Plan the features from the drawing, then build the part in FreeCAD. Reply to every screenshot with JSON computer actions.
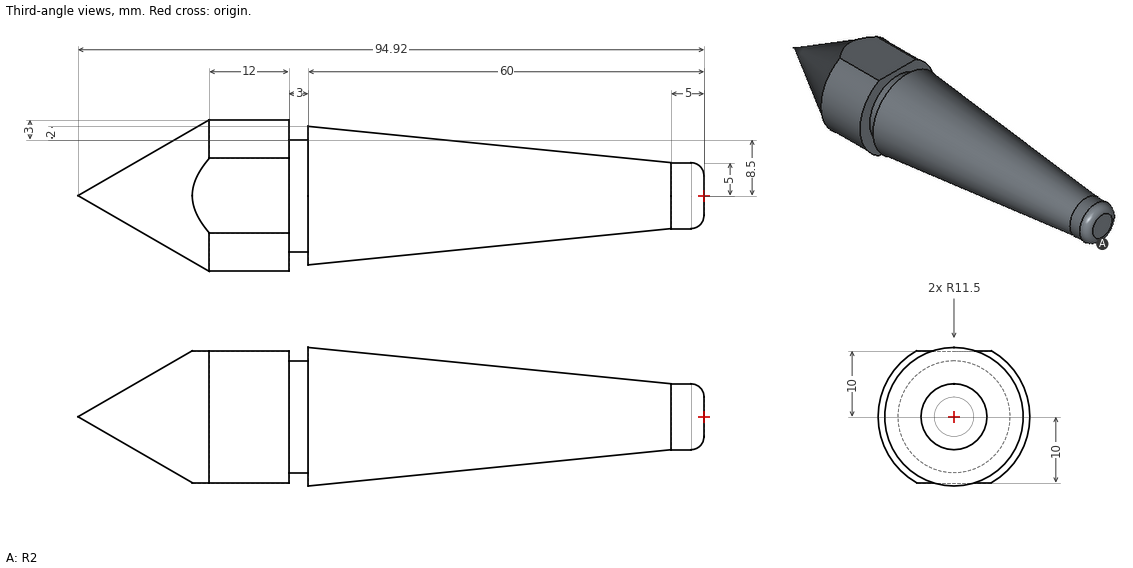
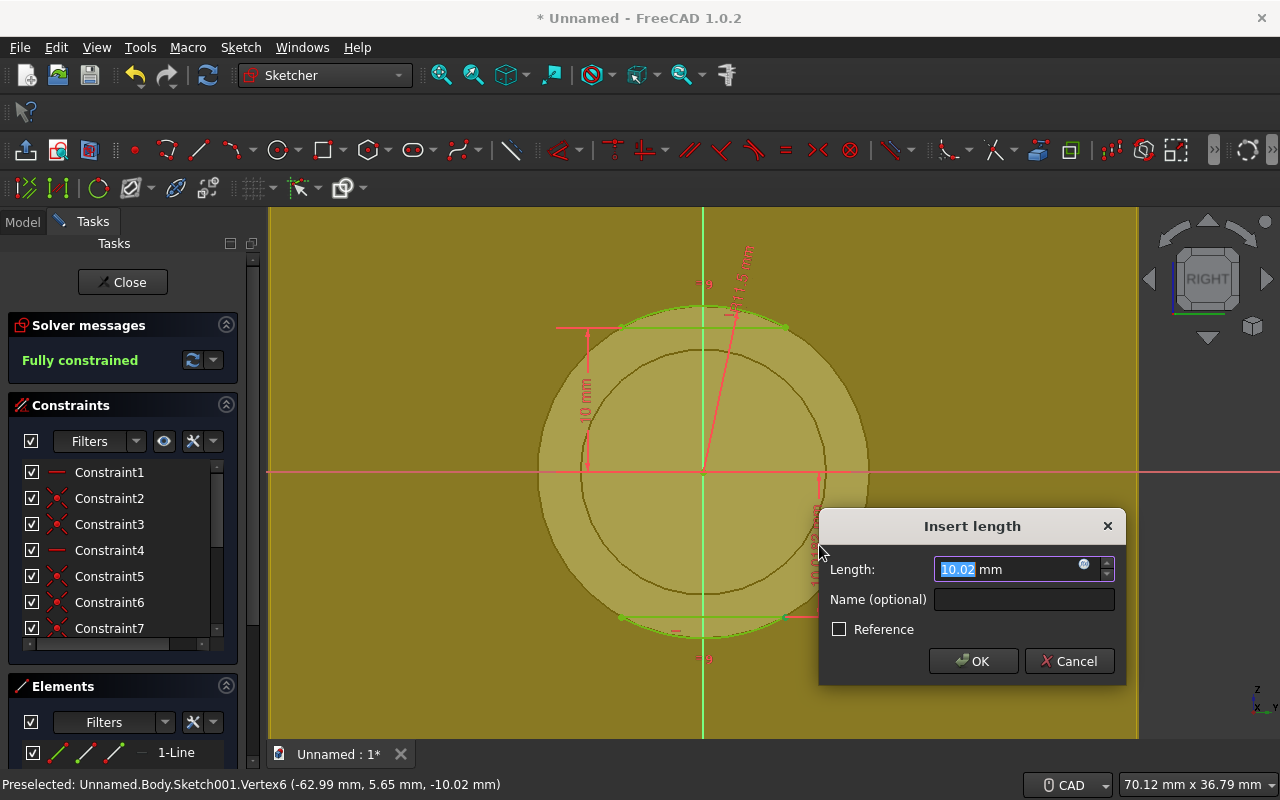
{"action": "type", "text": "10"}
{"action": "key", "text": "Return"}
{"action": "key", "text": "Escape"}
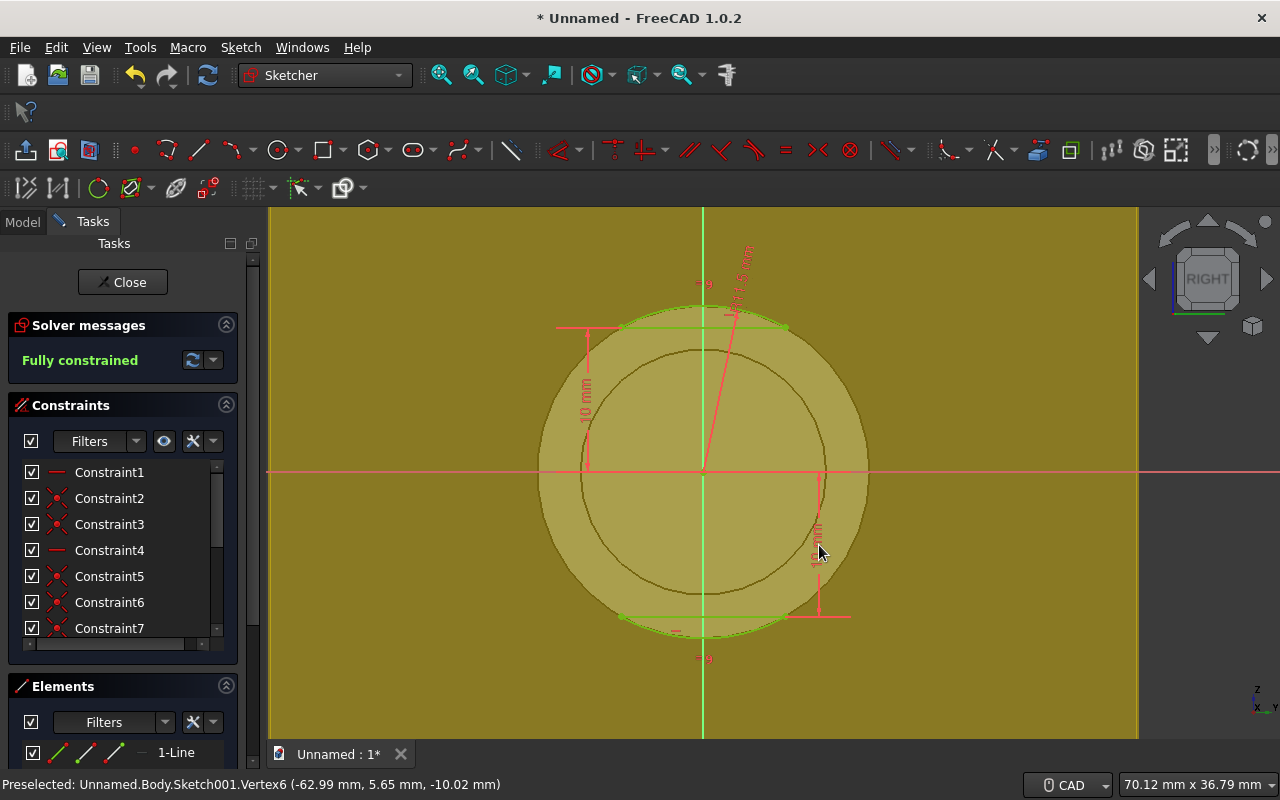
{"action": "left_click", "coordinate": [123, 282]}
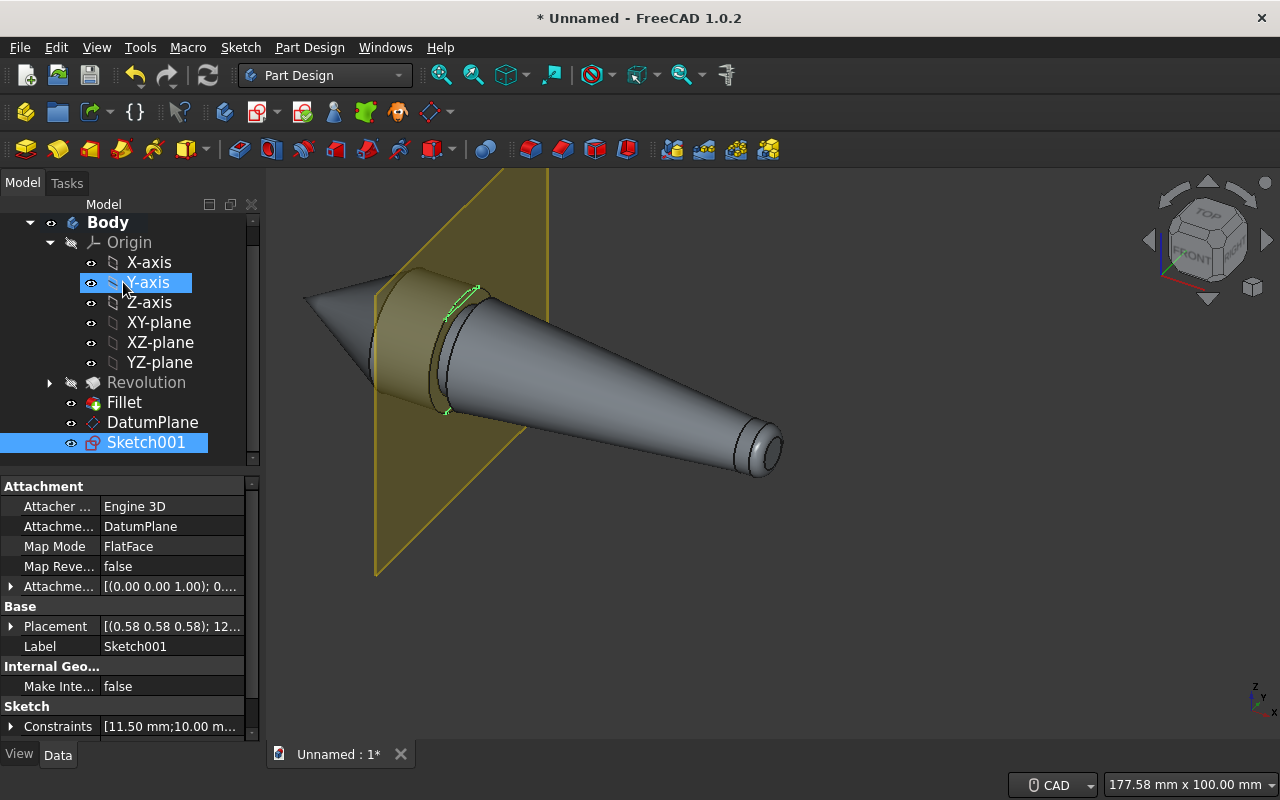
{"action": "left_click", "coordinate": [240, 150]}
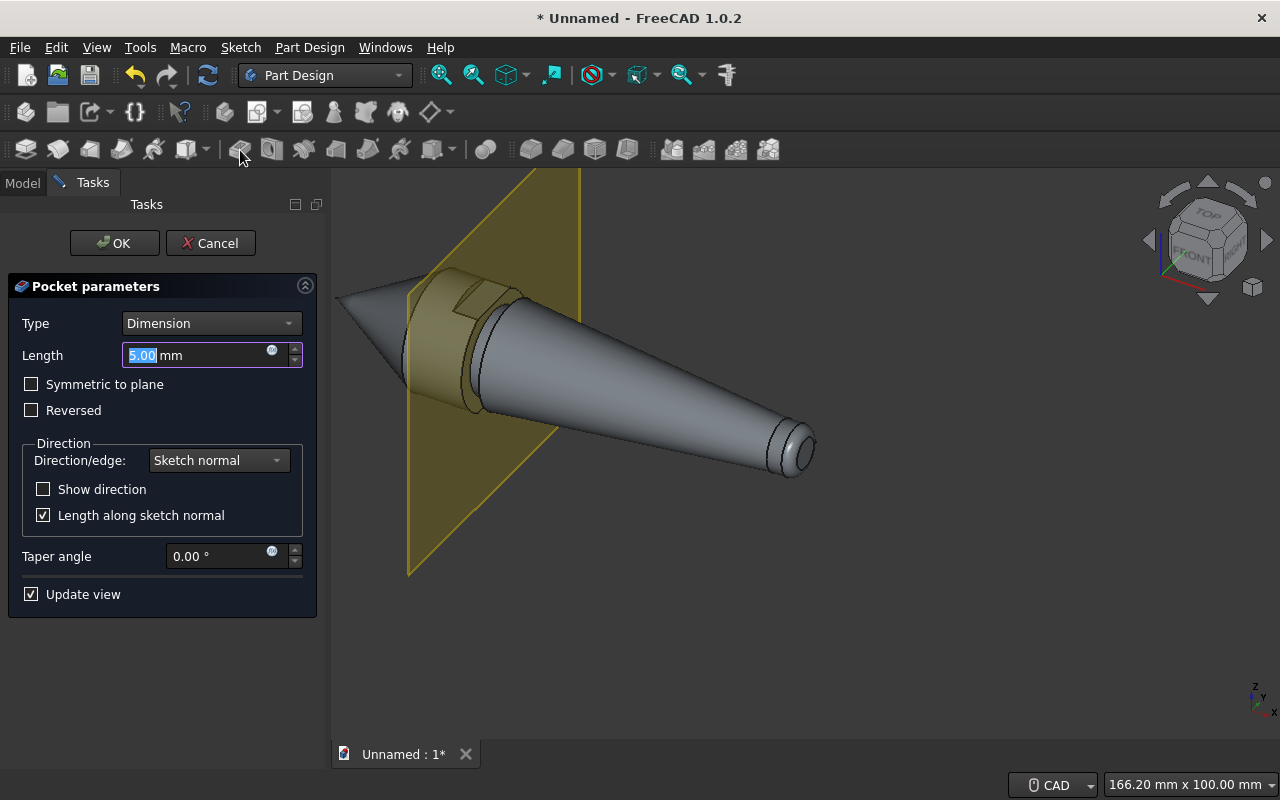
{"action": "left_click", "coordinate": [212, 324]}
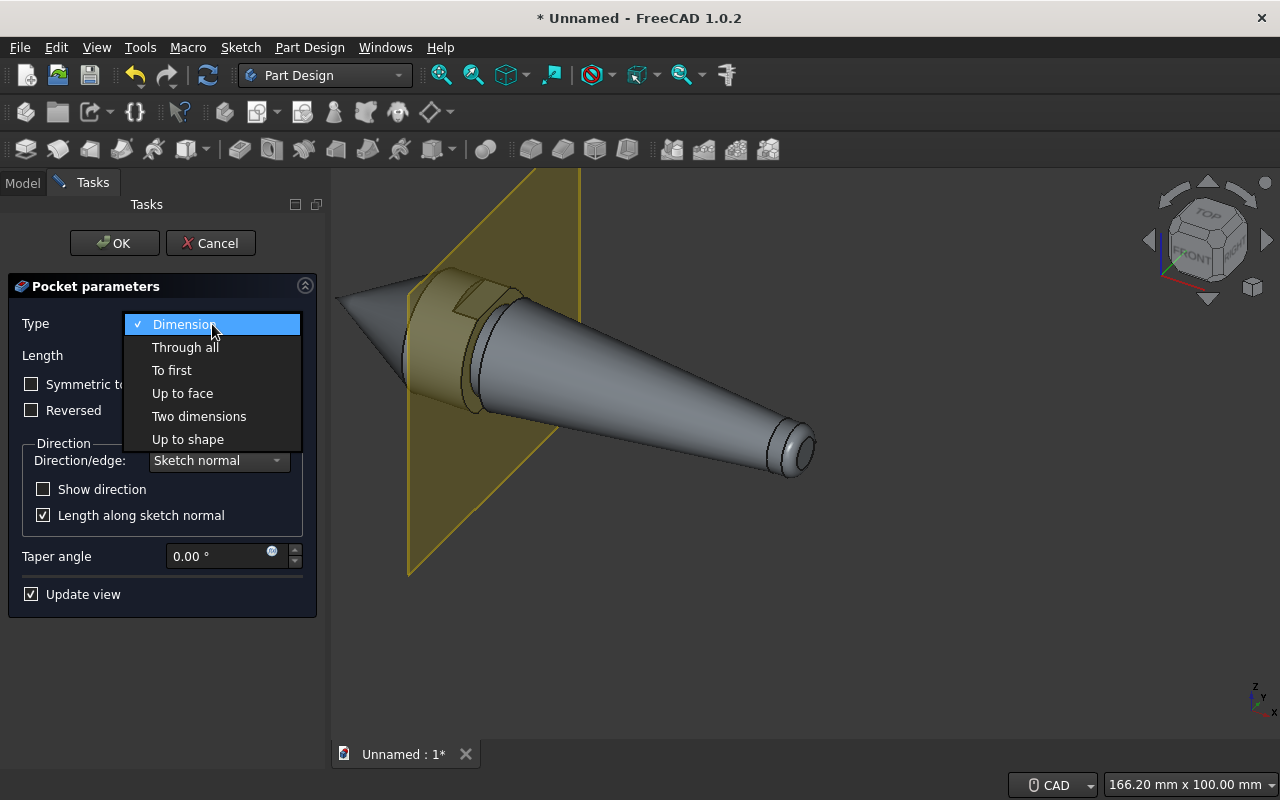
{"action": "left_click", "coordinate": [212, 348]}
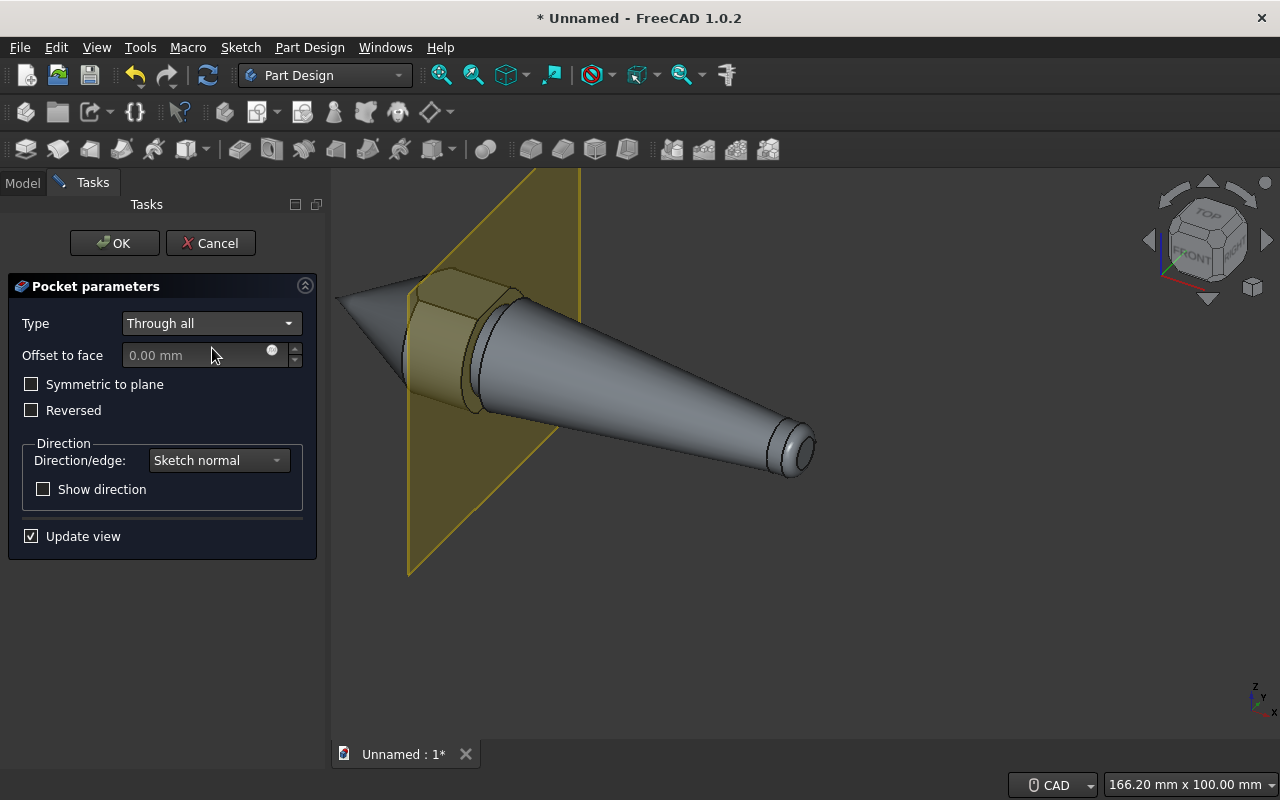
{"action": "left_click", "coordinate": [115, 243]}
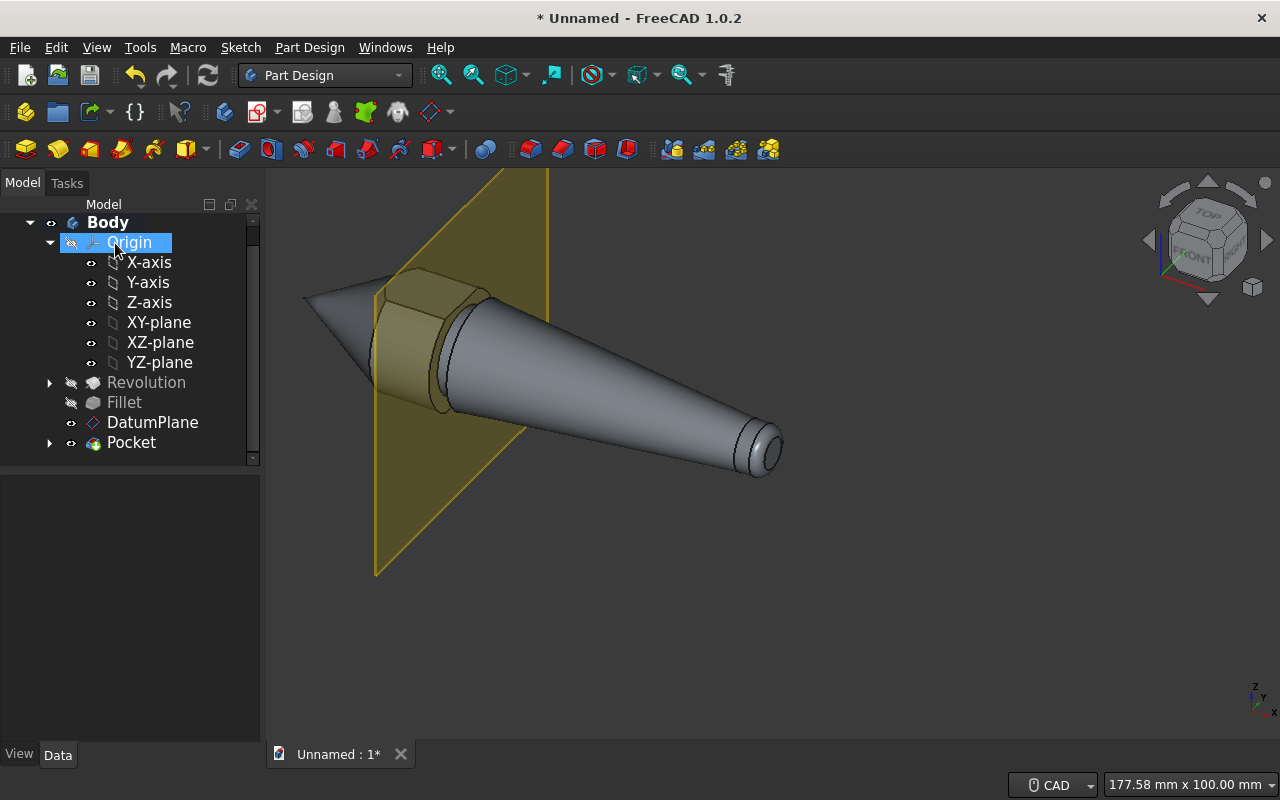
{"action": "left_click", "coordinate": [116, 423]}
{"action": "key", "text": "space"}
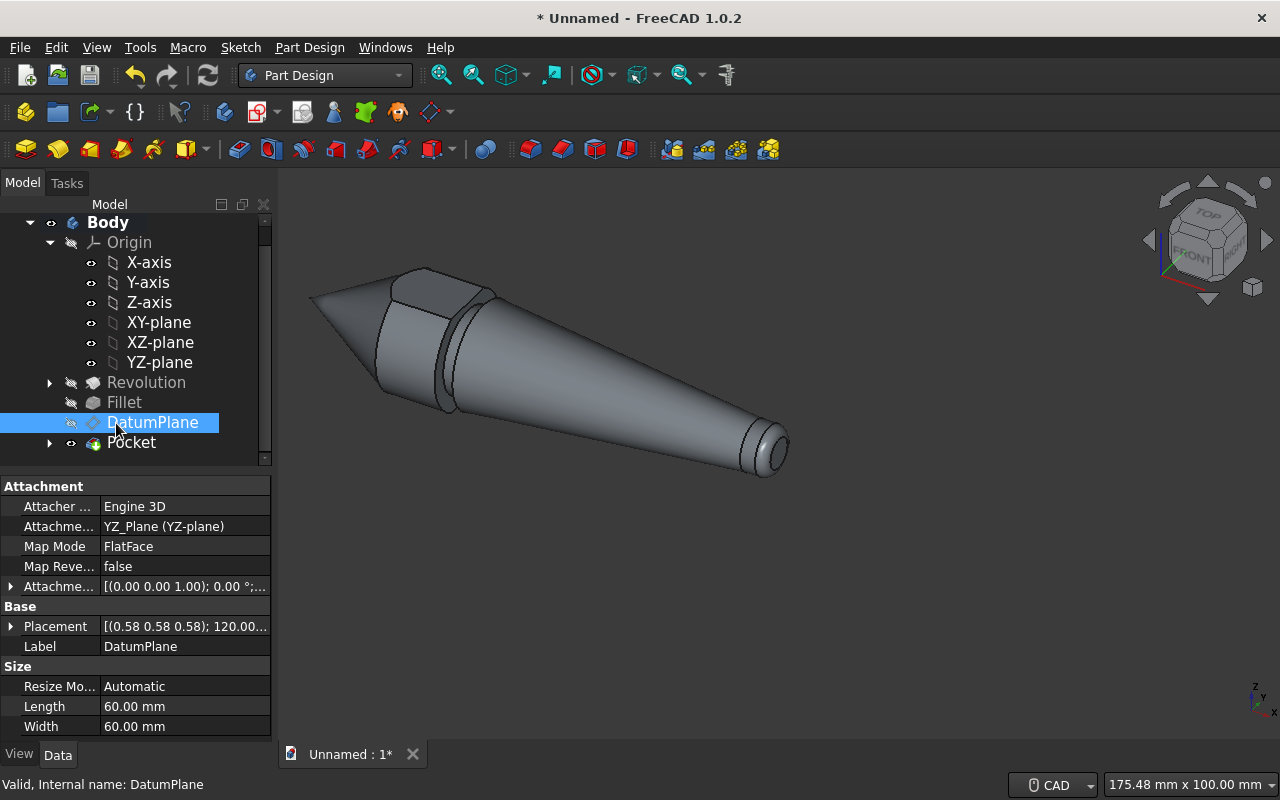
{"action": "key", "text": "0"}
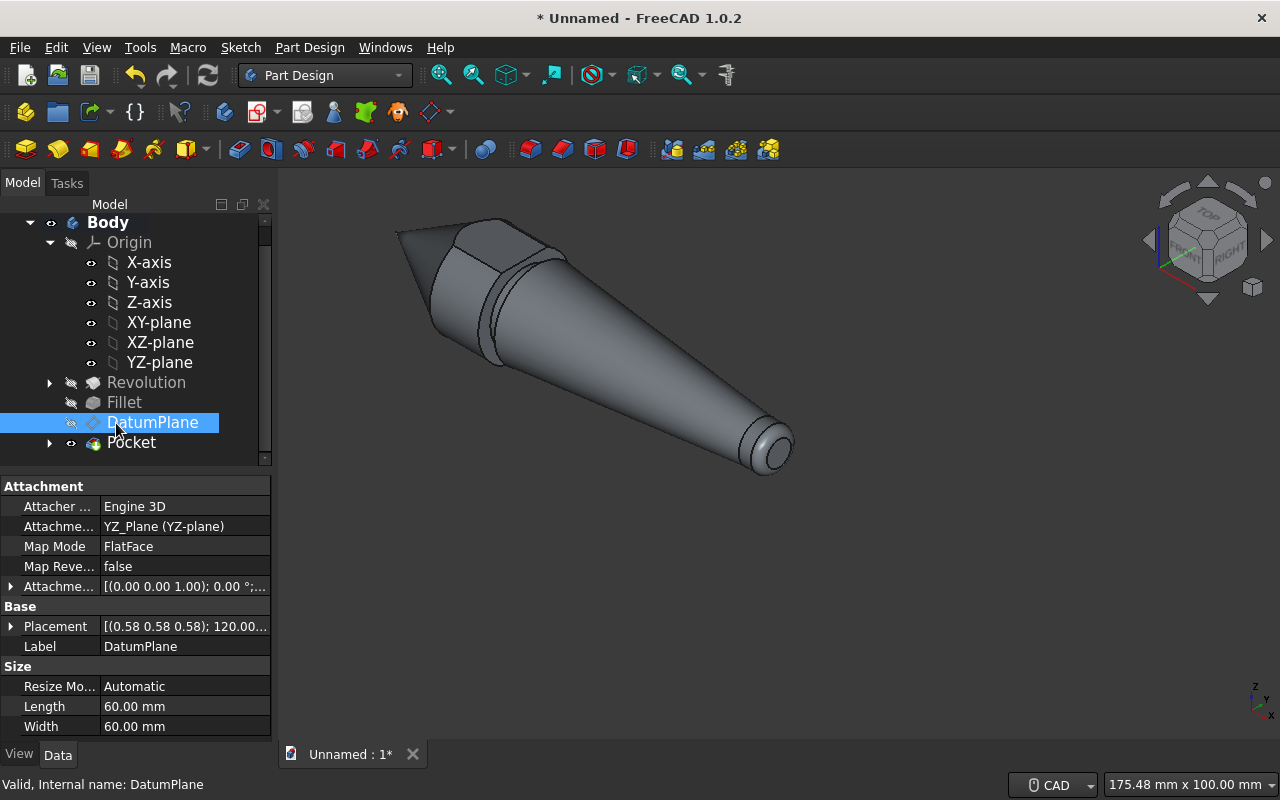
{"action": "left_click", "coordinate": [442, 76]}